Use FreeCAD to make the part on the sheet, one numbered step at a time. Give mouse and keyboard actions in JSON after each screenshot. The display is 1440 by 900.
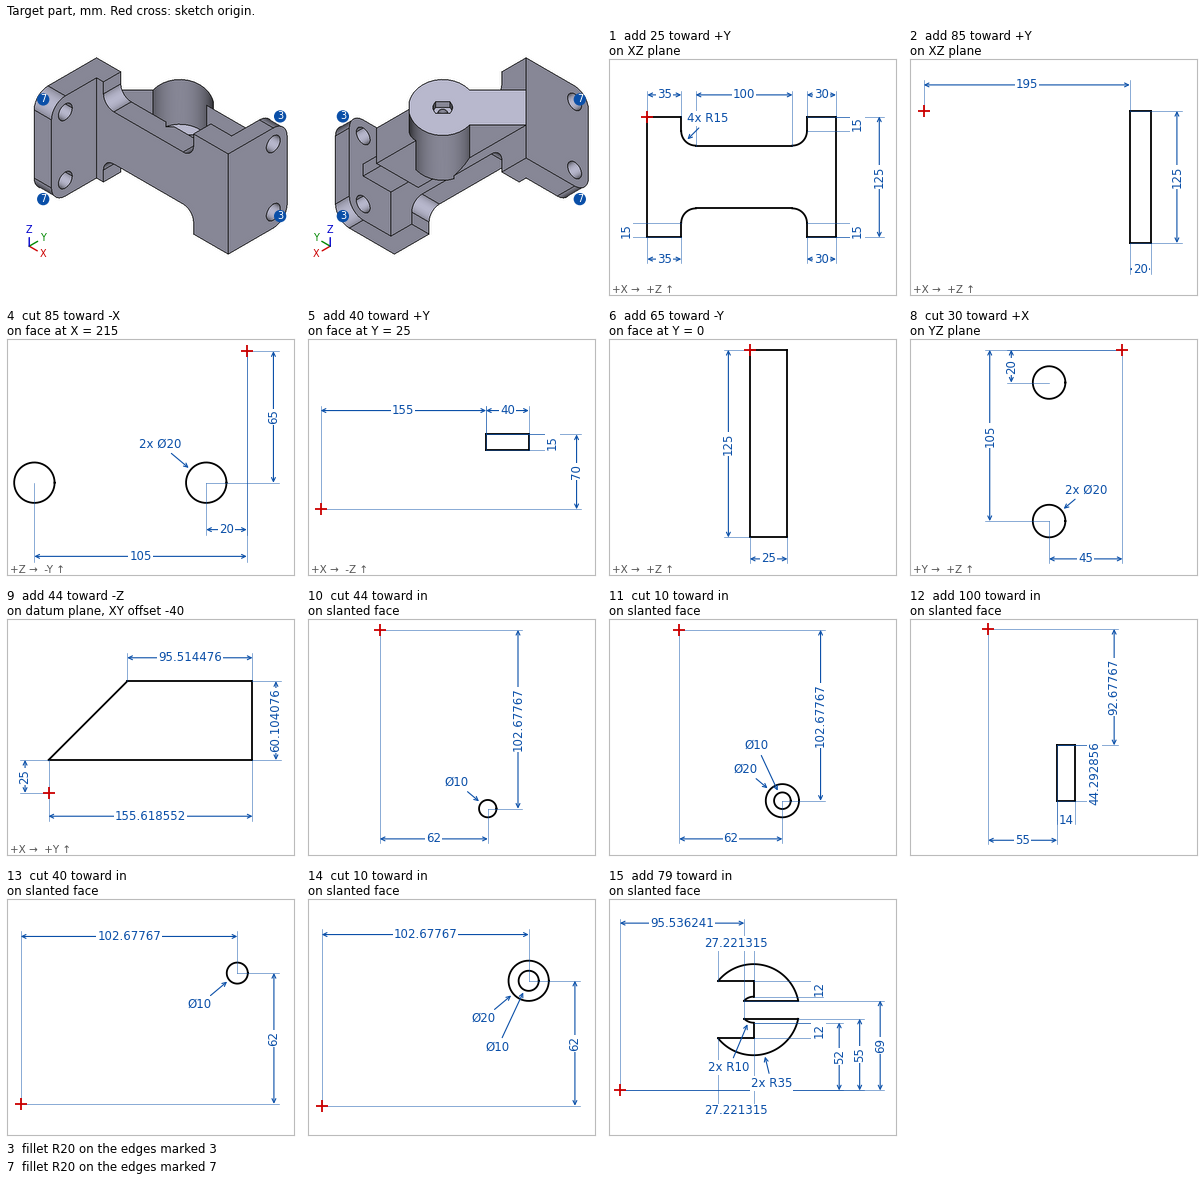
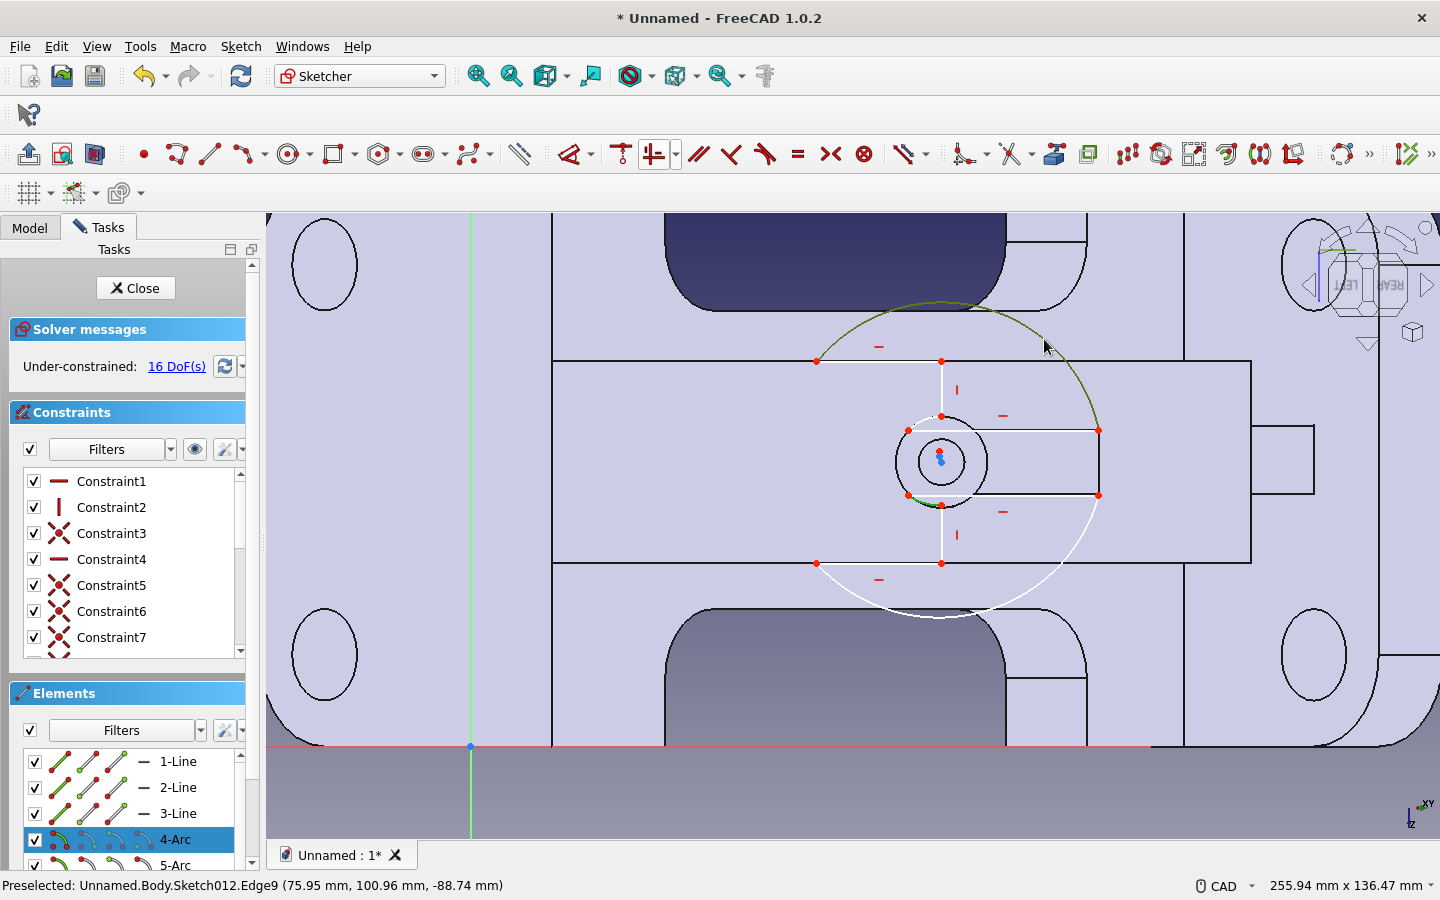
{"action": "left_click", "coordinate": [621, 154]}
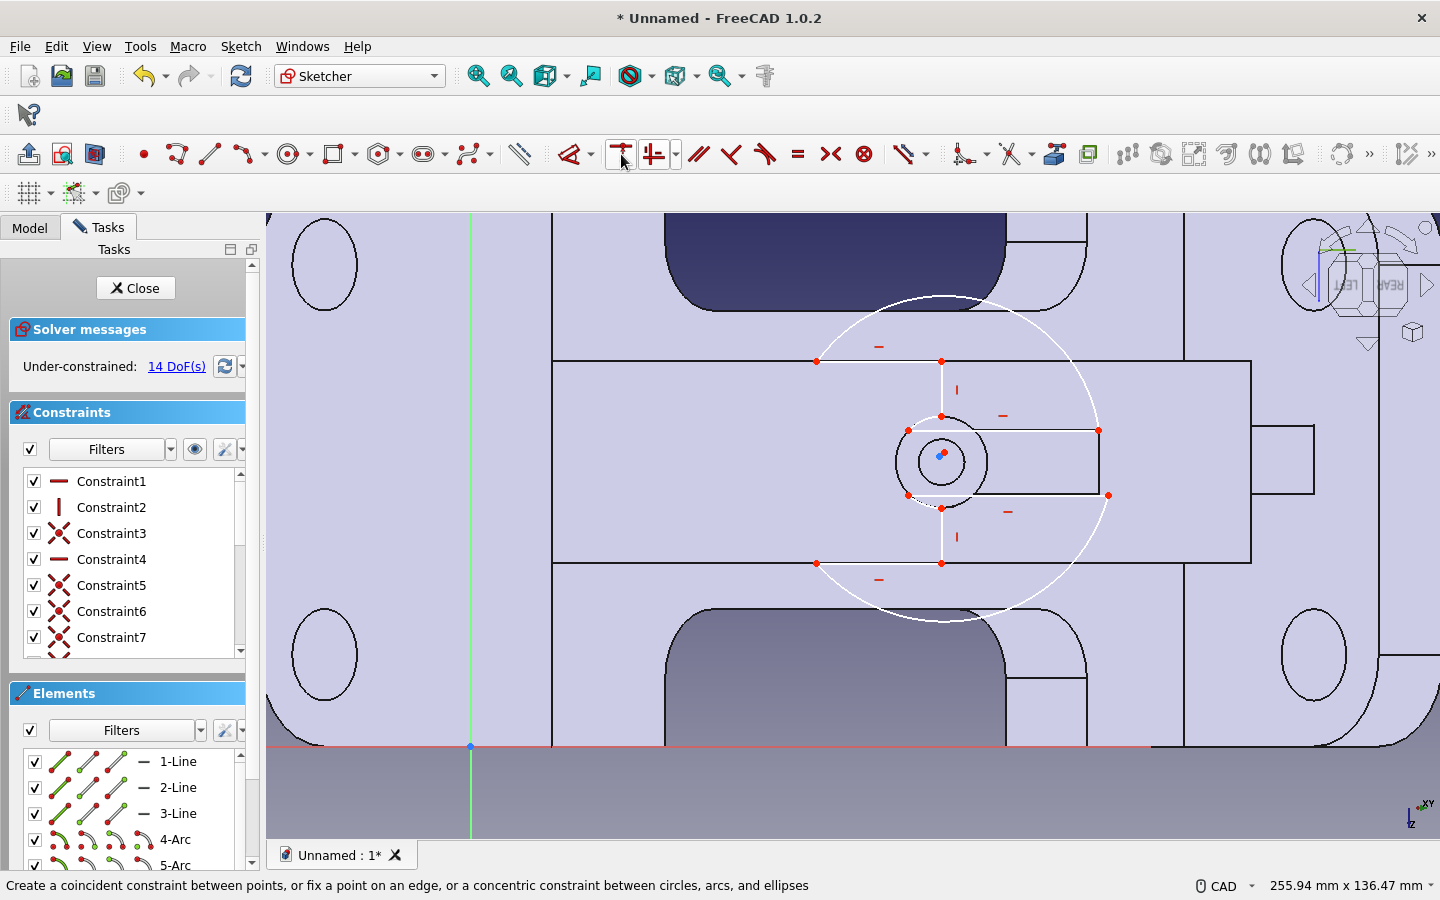
{"action": "scroll", "coordinate": [931, 507], "scroll_direction": "up", "scroll_amount": 2}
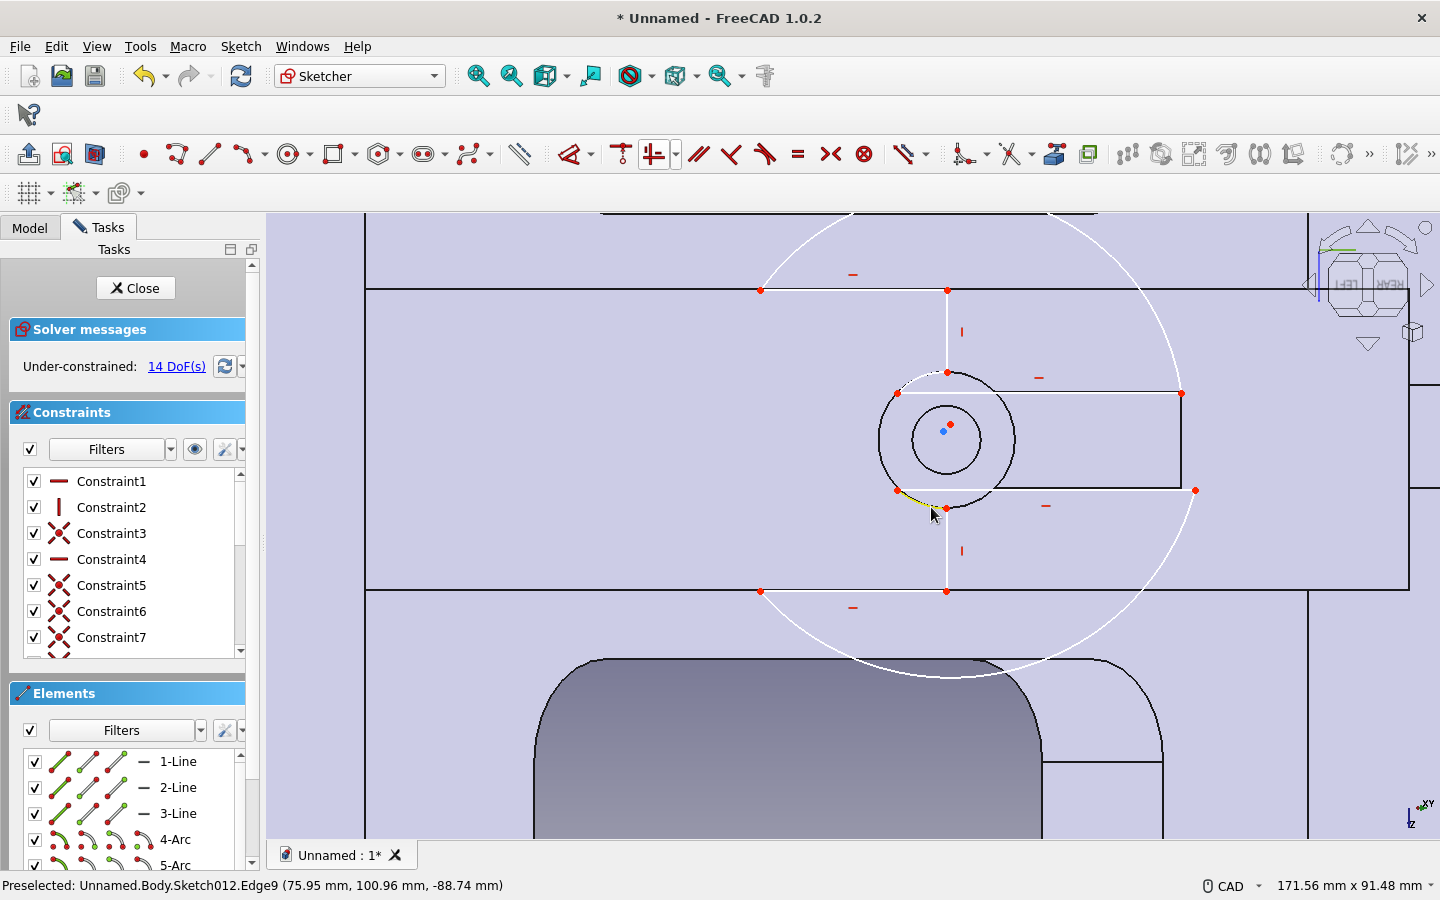
{"action": "left_click", "coordinate": [931, 507]}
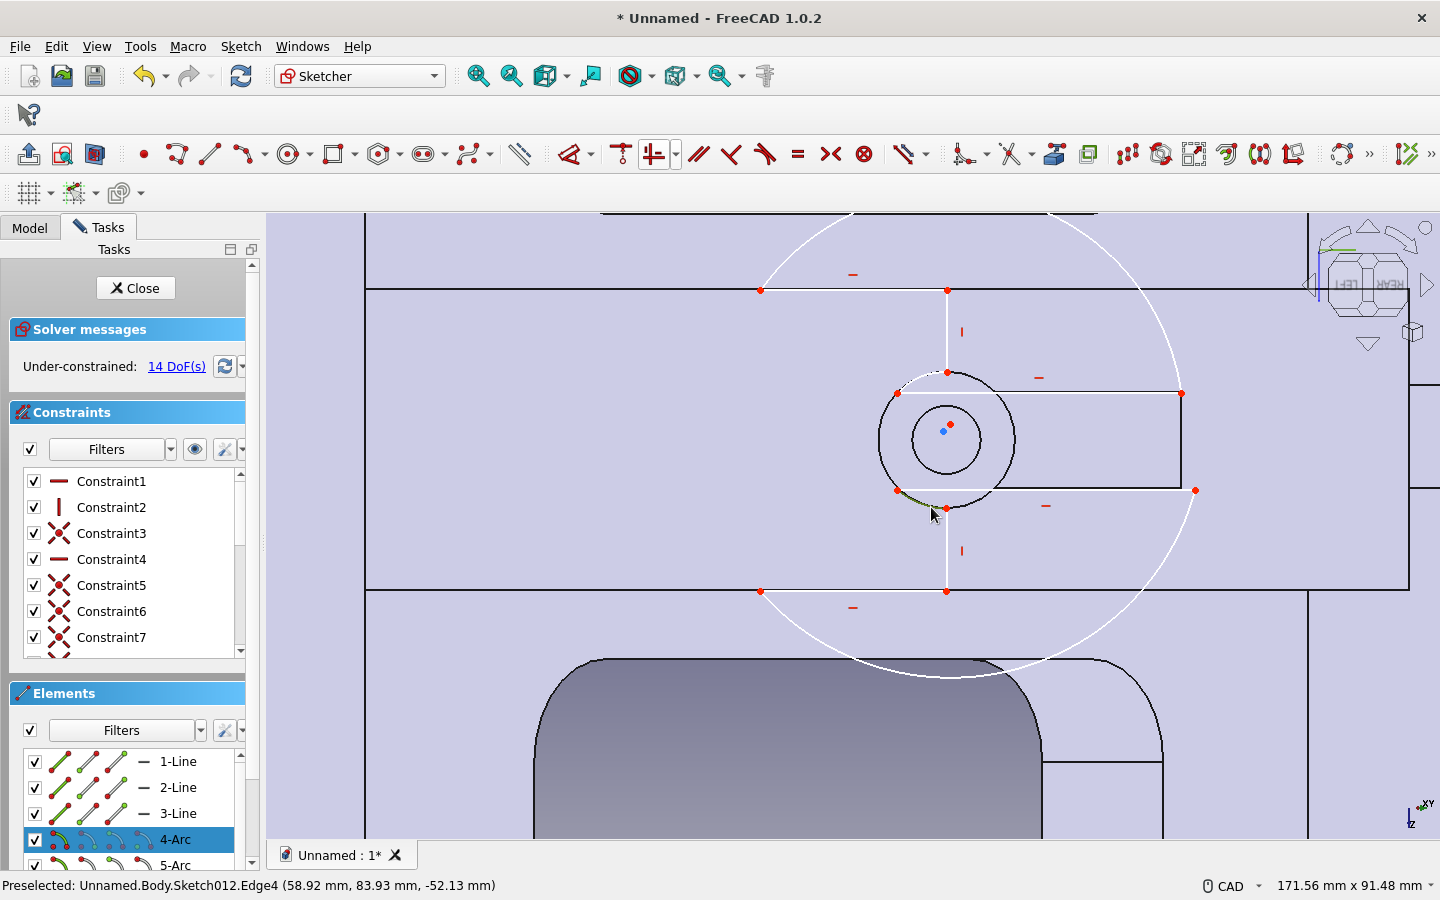
{"action": "left_click", "coordinate": [931, 374]}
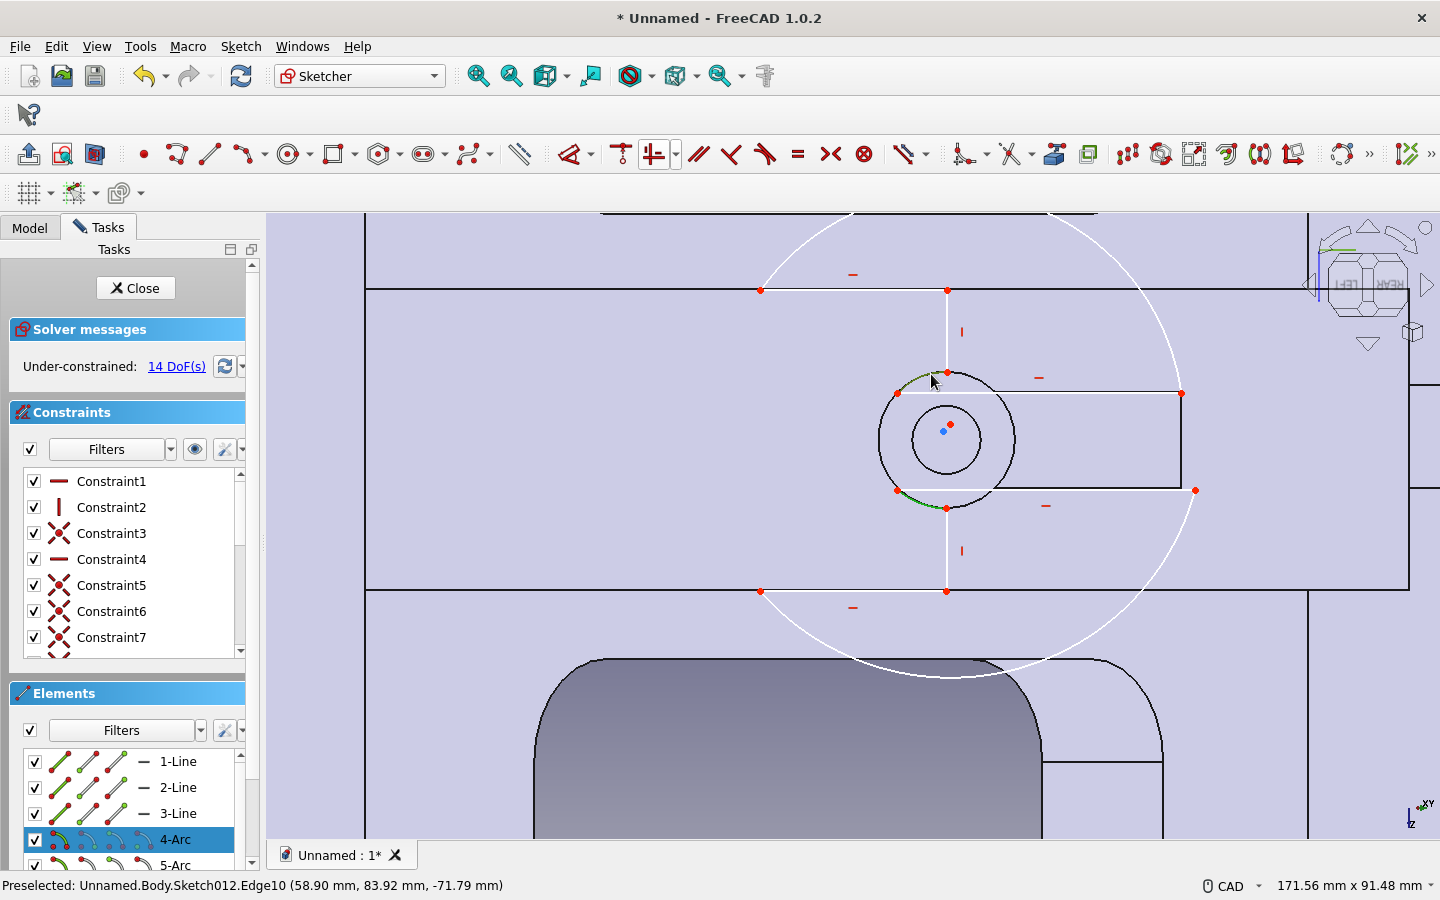
{"action": "left_click", "coordinate": [621, 154]}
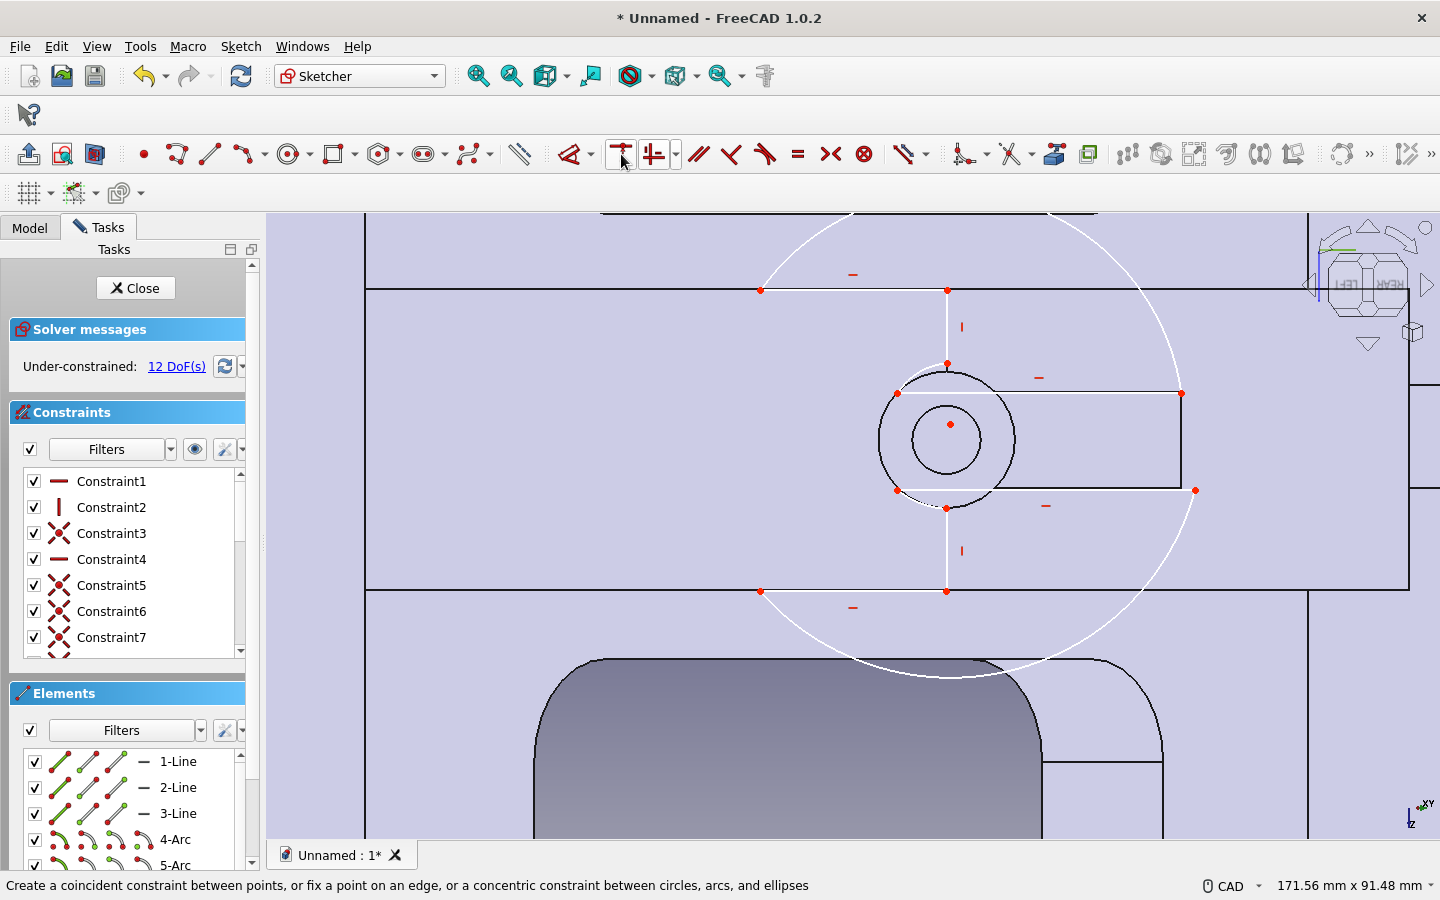
{"action": "left_click", "coordinate": [900, 673]}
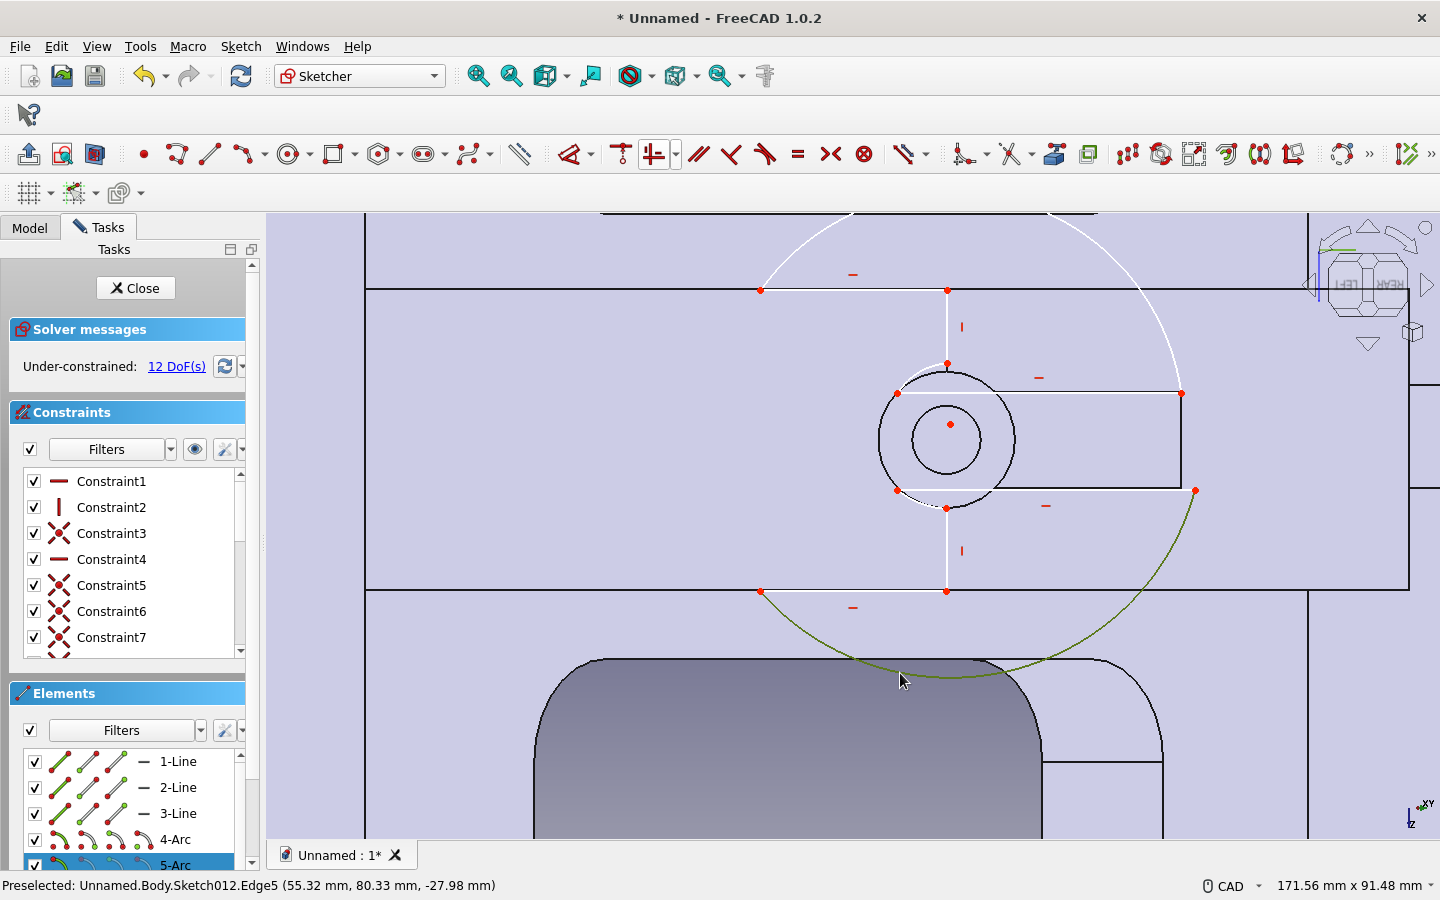
{"action": "left_click", "coordinate": [1104, 250]}